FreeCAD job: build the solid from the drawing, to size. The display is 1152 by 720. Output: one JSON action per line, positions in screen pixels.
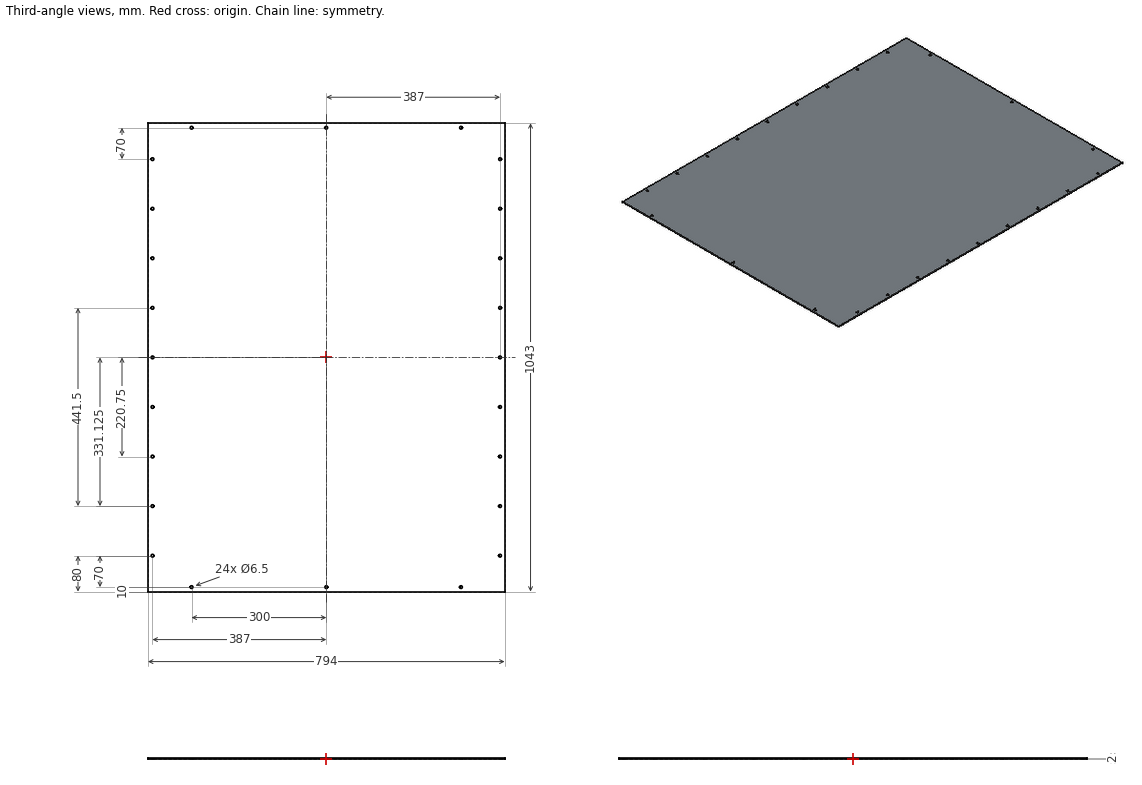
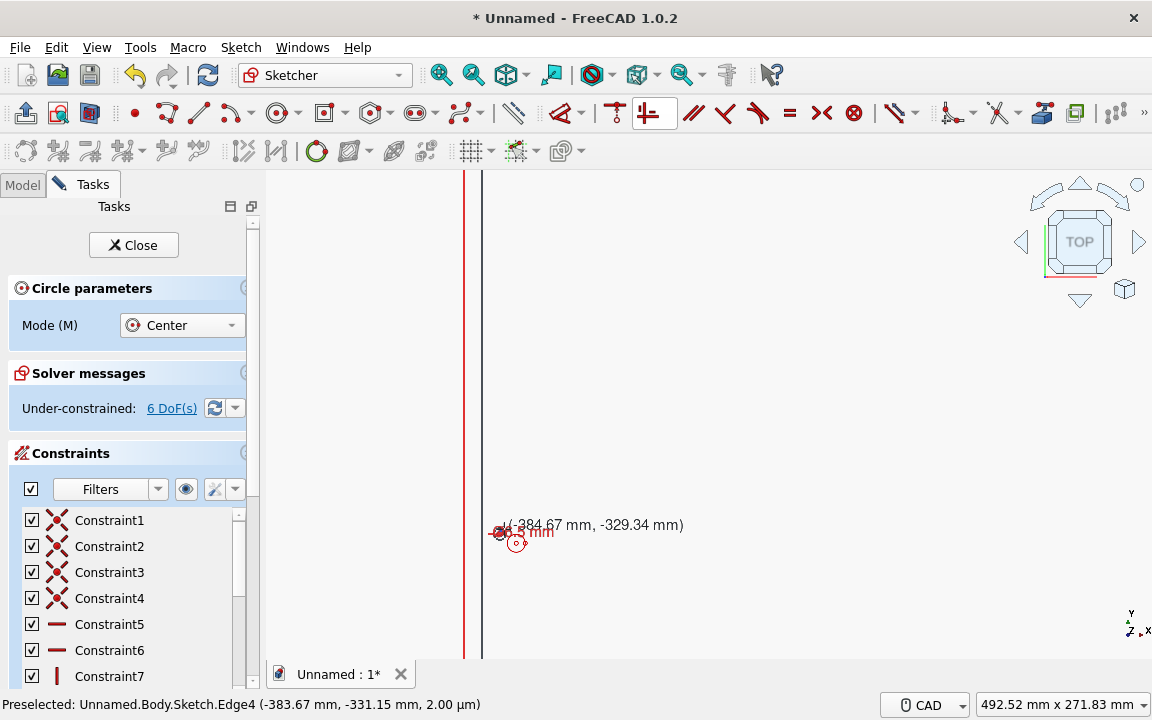
{"action": "scroll", "coordinate": [530, 509], "scroll_direction": "down", "scroll_amount": 9}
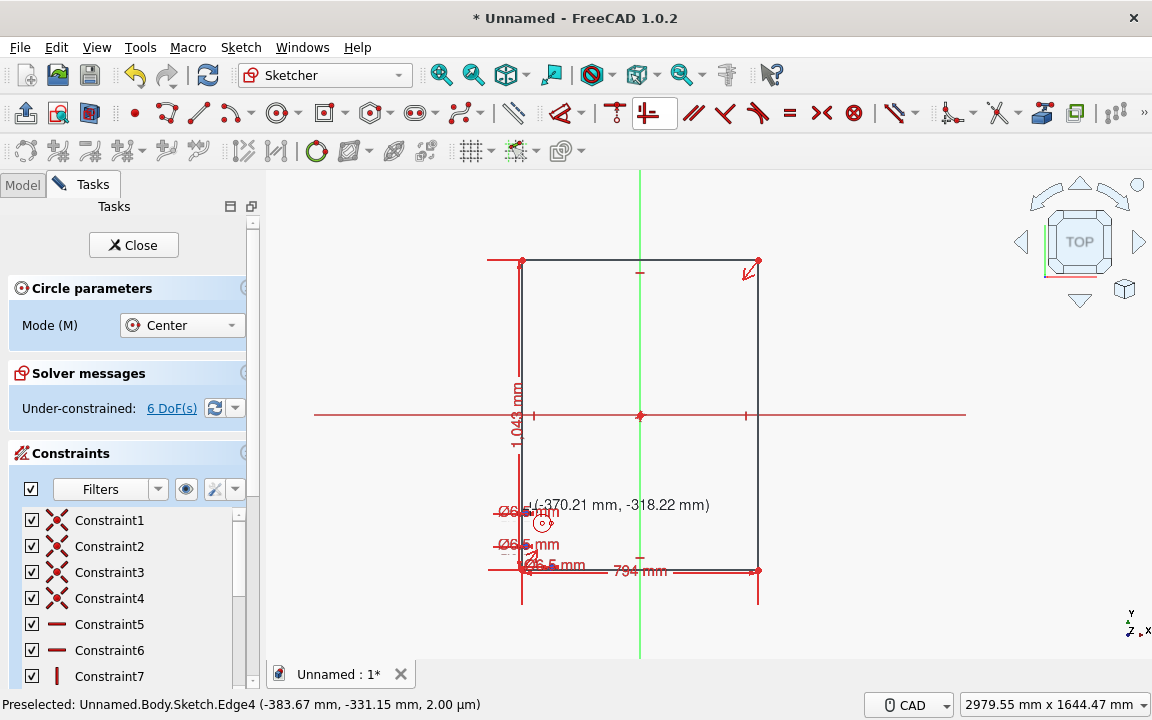
{"action": "scroll", "coordinate": [640, 567], "scroll_direction": "up", "scroll_amount": 16}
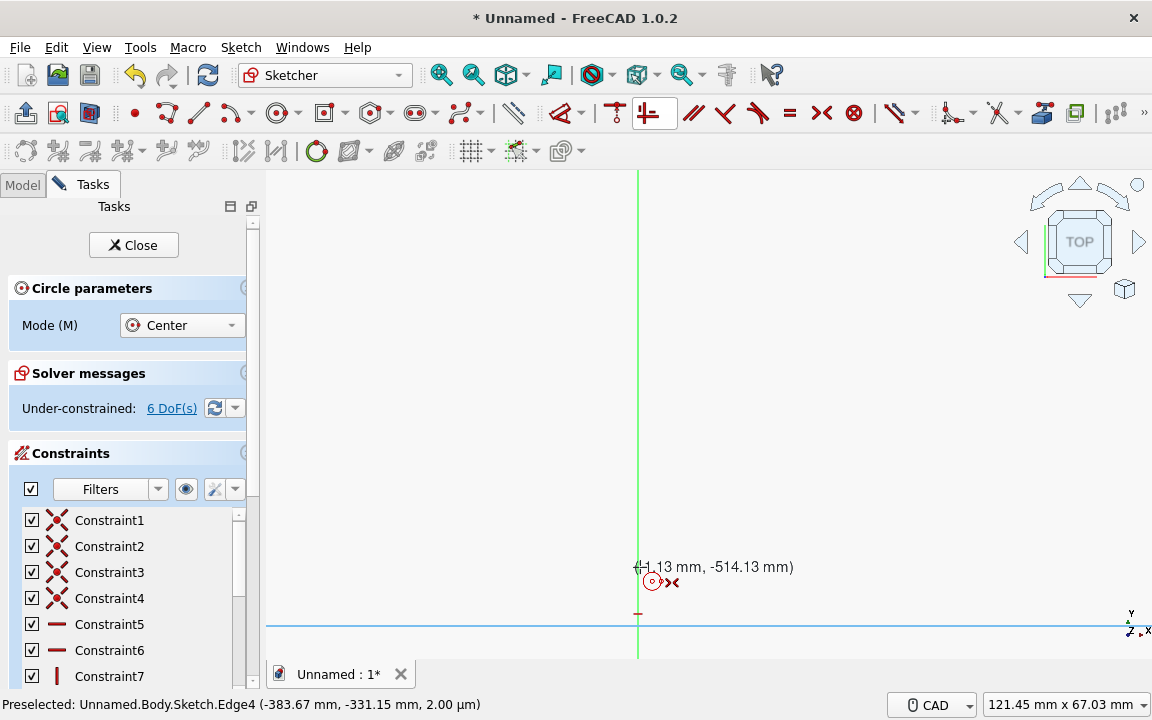
{"action": "scroll", "coordinate": [641, 603], "scroll_direction": "down", "scroll_amount": 15}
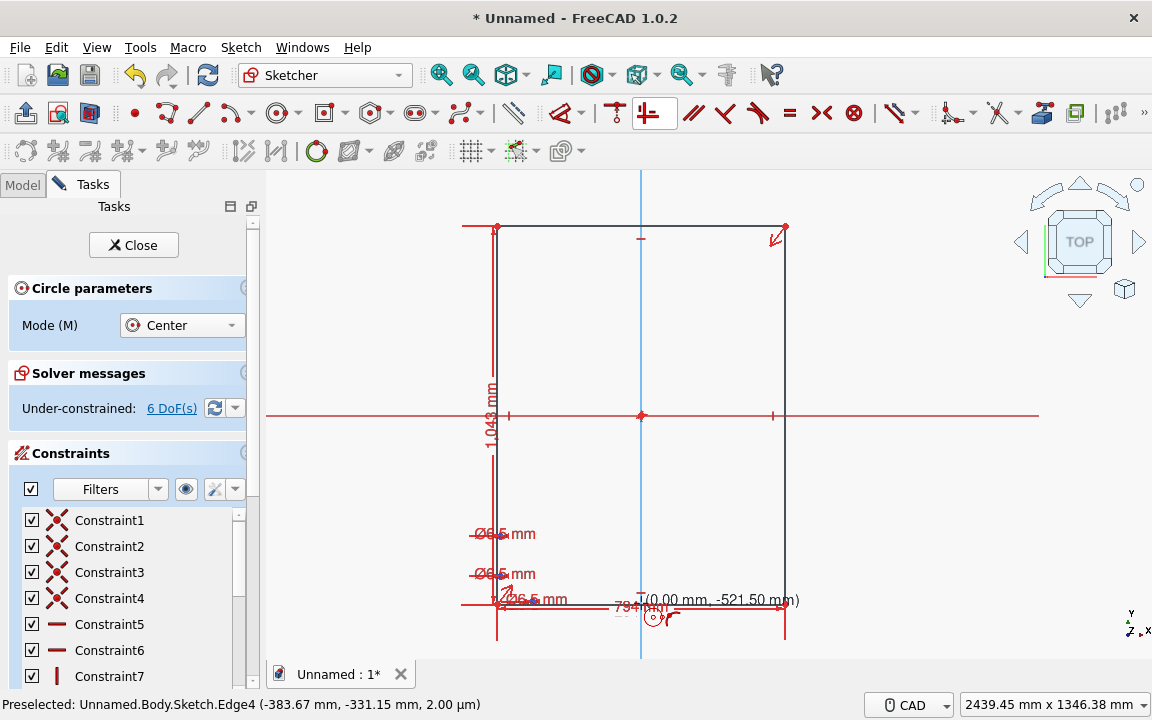
{"action": "scroll", "coordinate": [641, 601], "scroll_direction": "up", "scroll_amount": 8}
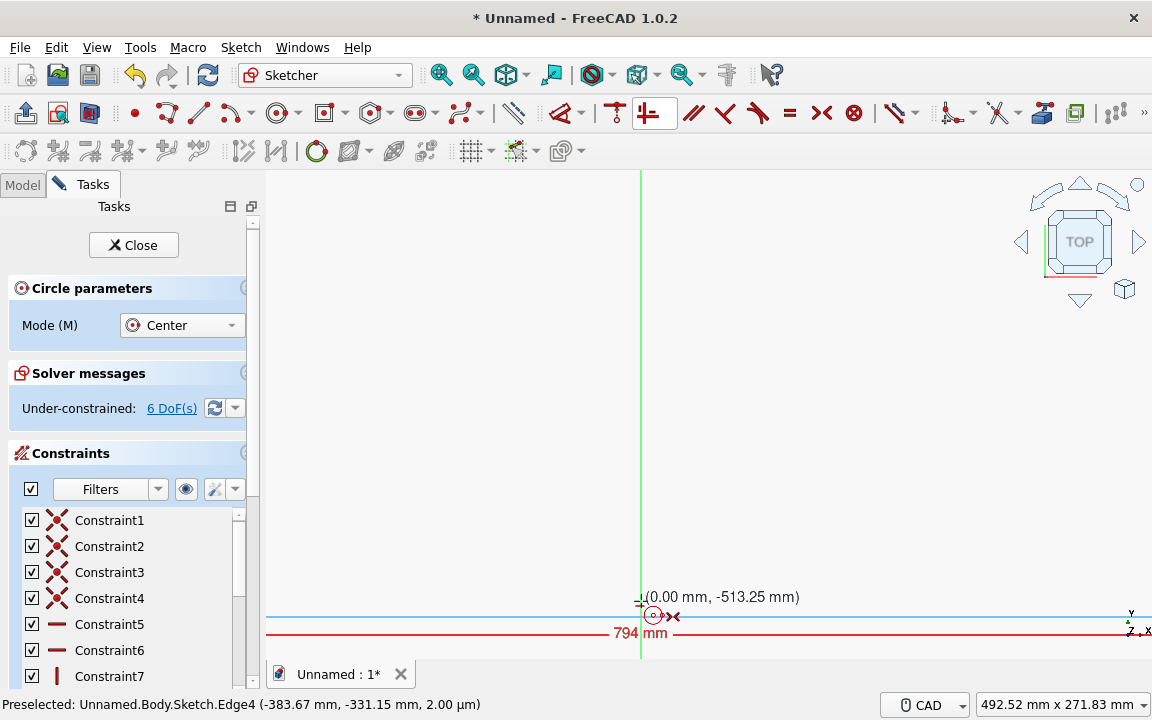
{"action": "left_click", "coordinate": [641, 599]}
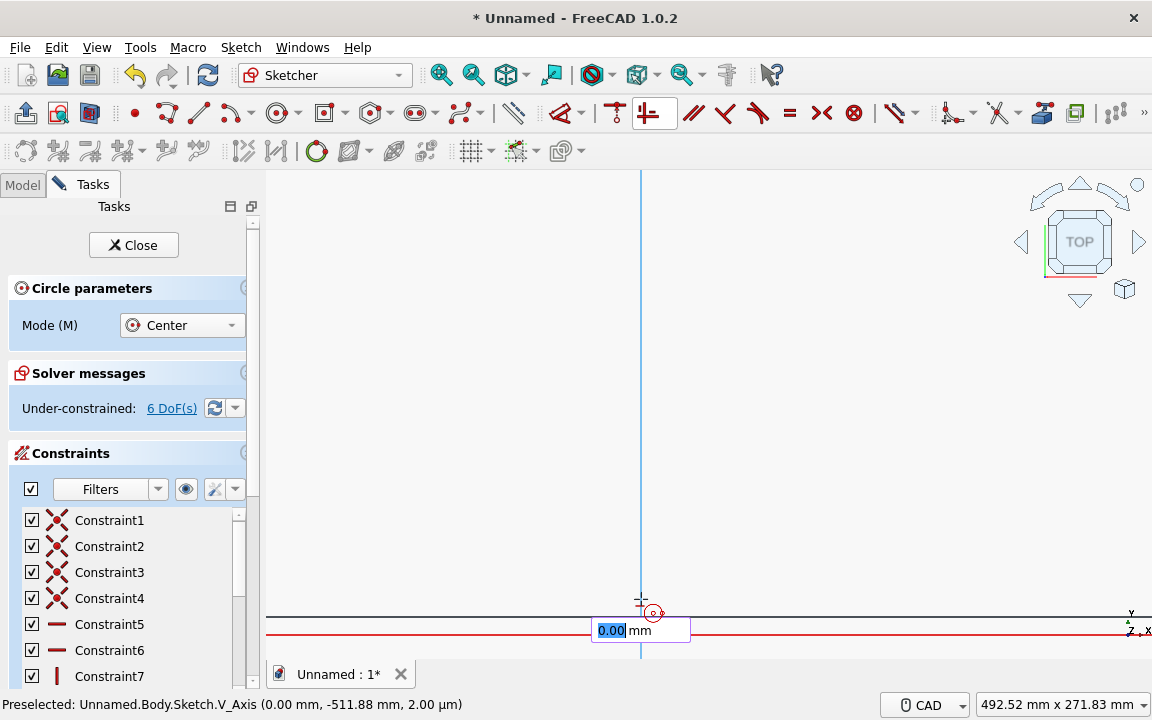
{"action": "scroll", "coordinate": [646, 597], "scroll_direction": "up", "scroll_amount": 6}
{"action": "mouse_move", "coordinate": [645, 596]}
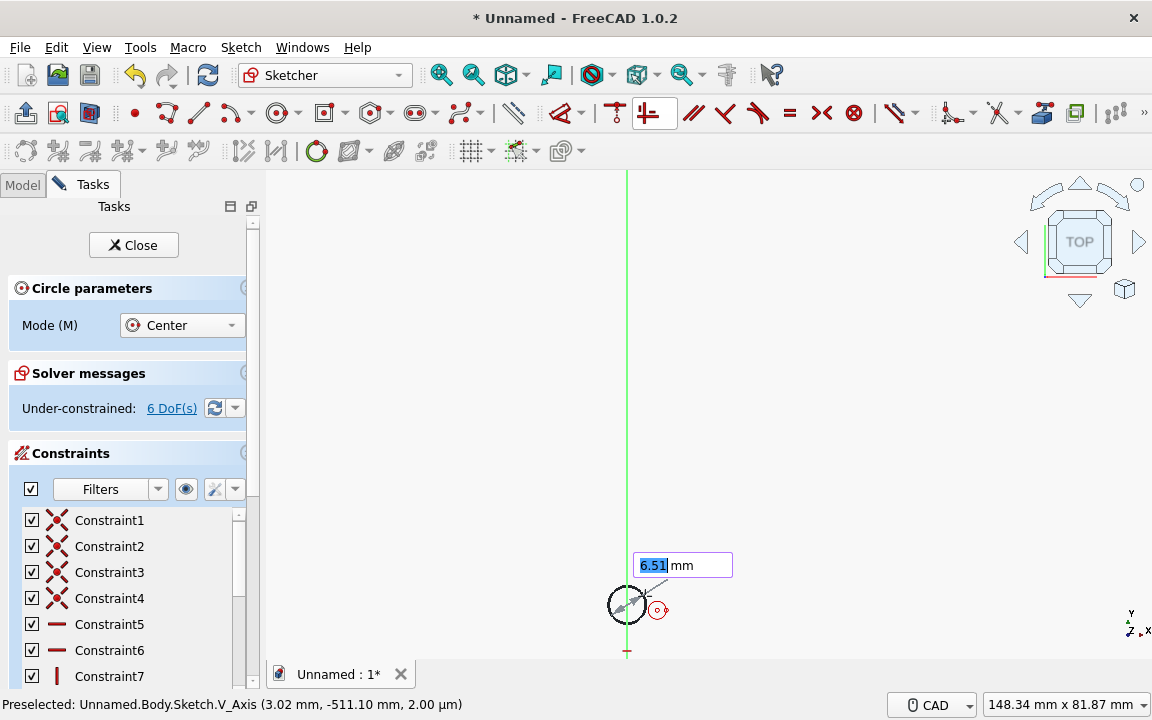
{"action": "type", "text": "6.5"}
{"action": "key", "text": "Return"}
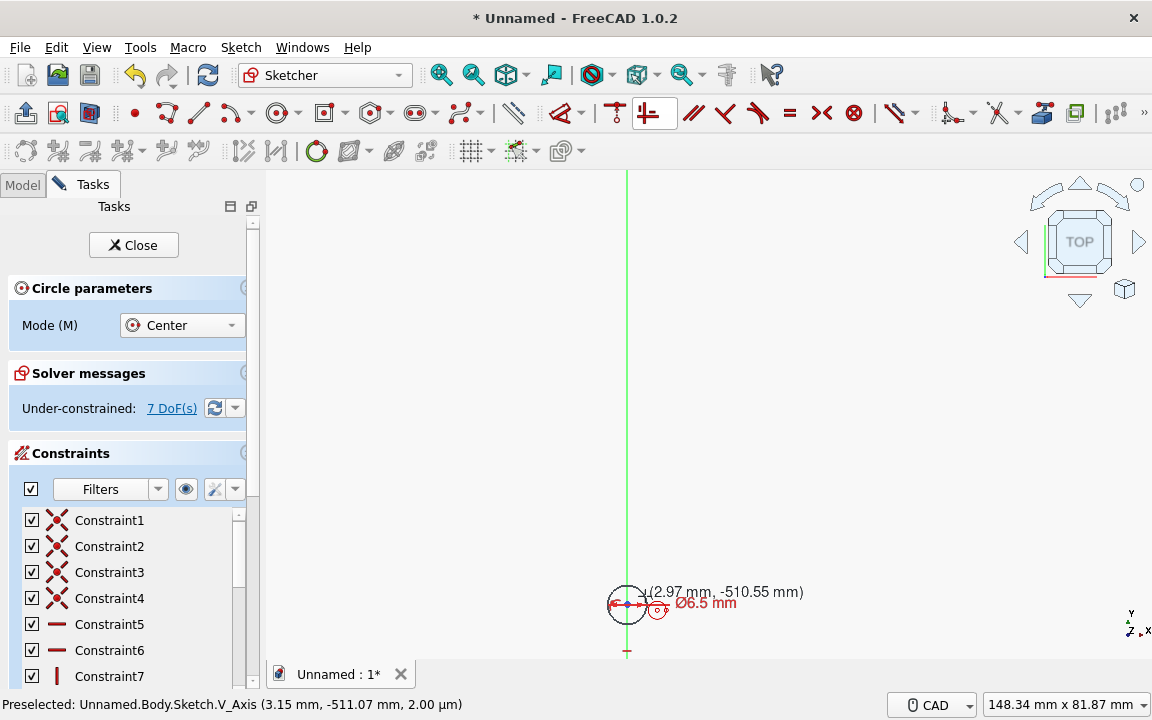
{"action": "scroll", "coordinate": [641, 565], "scroll_direction": "down", "scroll_amount": 15}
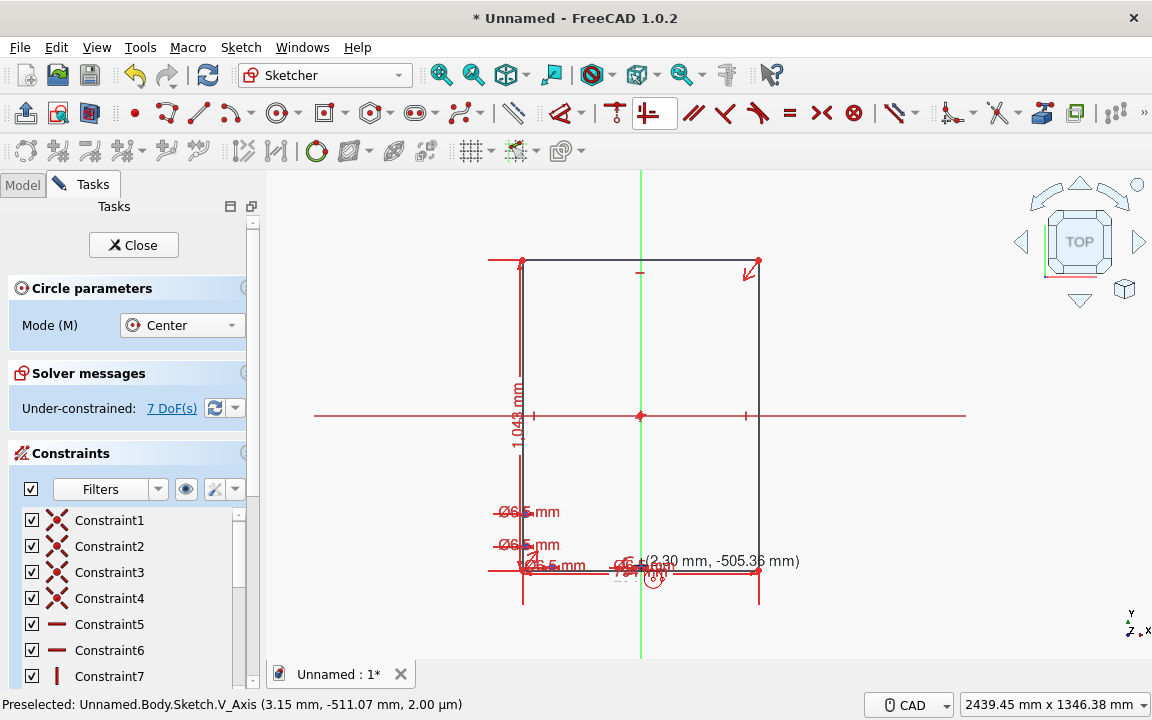
{"action": "scroll", "coordinate": [526, 481], "scroll_direction": "up", "scroll_amount": 16}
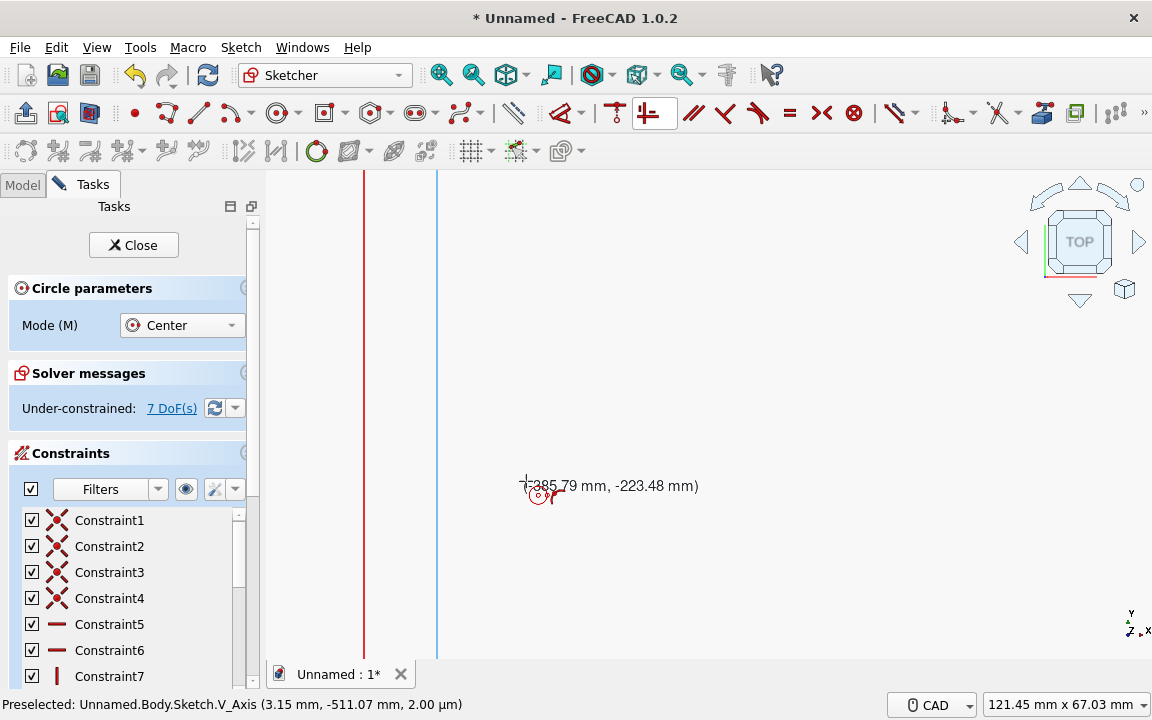
{"action": "scroll", "coordinate": [499, 496], "scroll_direction": "down", "scroll_amount": 15}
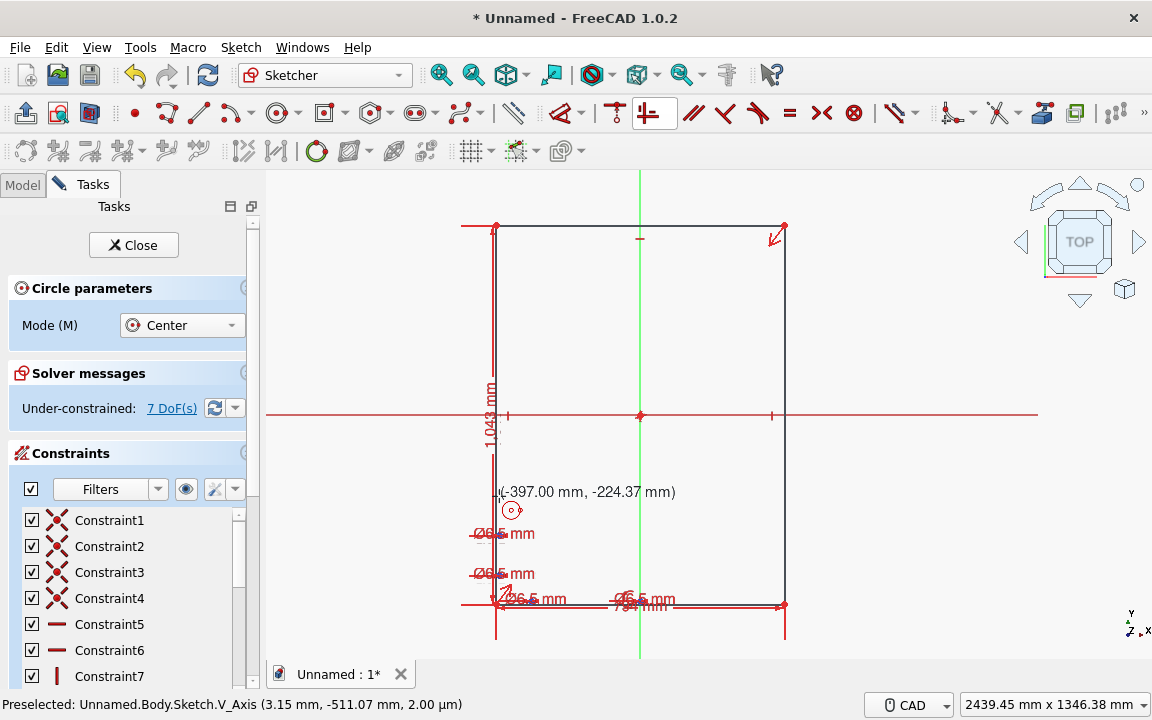
{"action": "scroll", "coordinate": [500, 495], "scroll_direction": "up", "scroll_amount": 8}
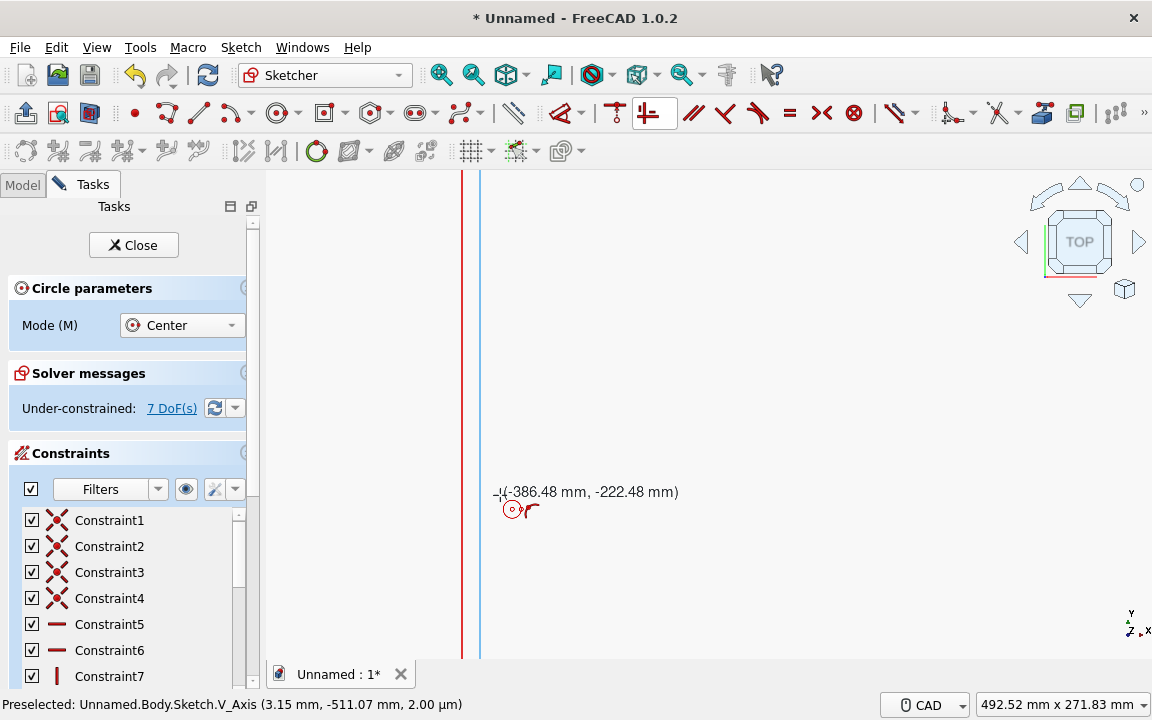
{"action": "left_click", "coordinate": [498, 494]}
{"action": "mouse_move", "coordinate": [502, 490]}